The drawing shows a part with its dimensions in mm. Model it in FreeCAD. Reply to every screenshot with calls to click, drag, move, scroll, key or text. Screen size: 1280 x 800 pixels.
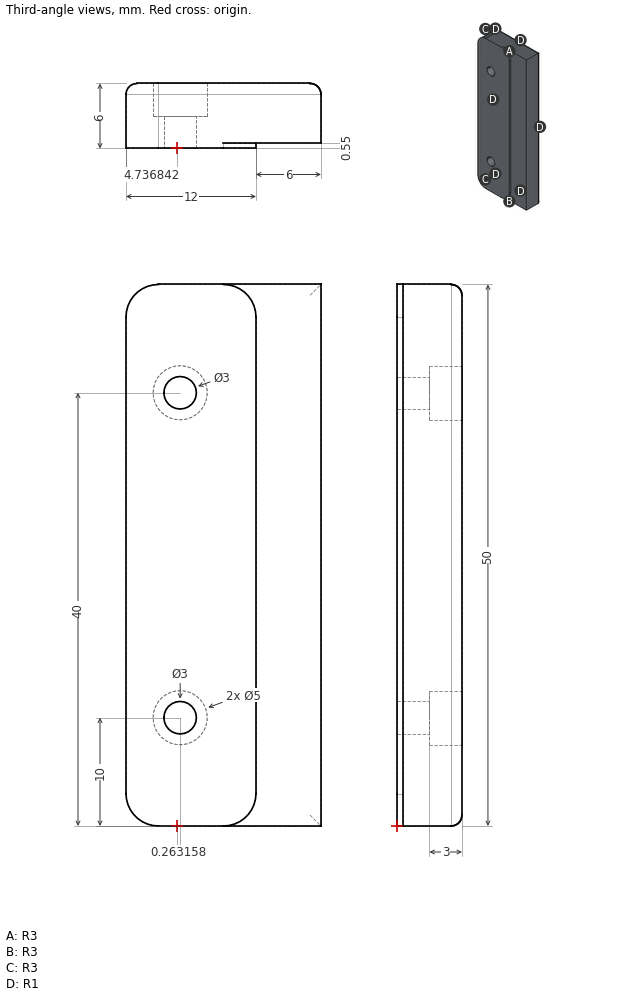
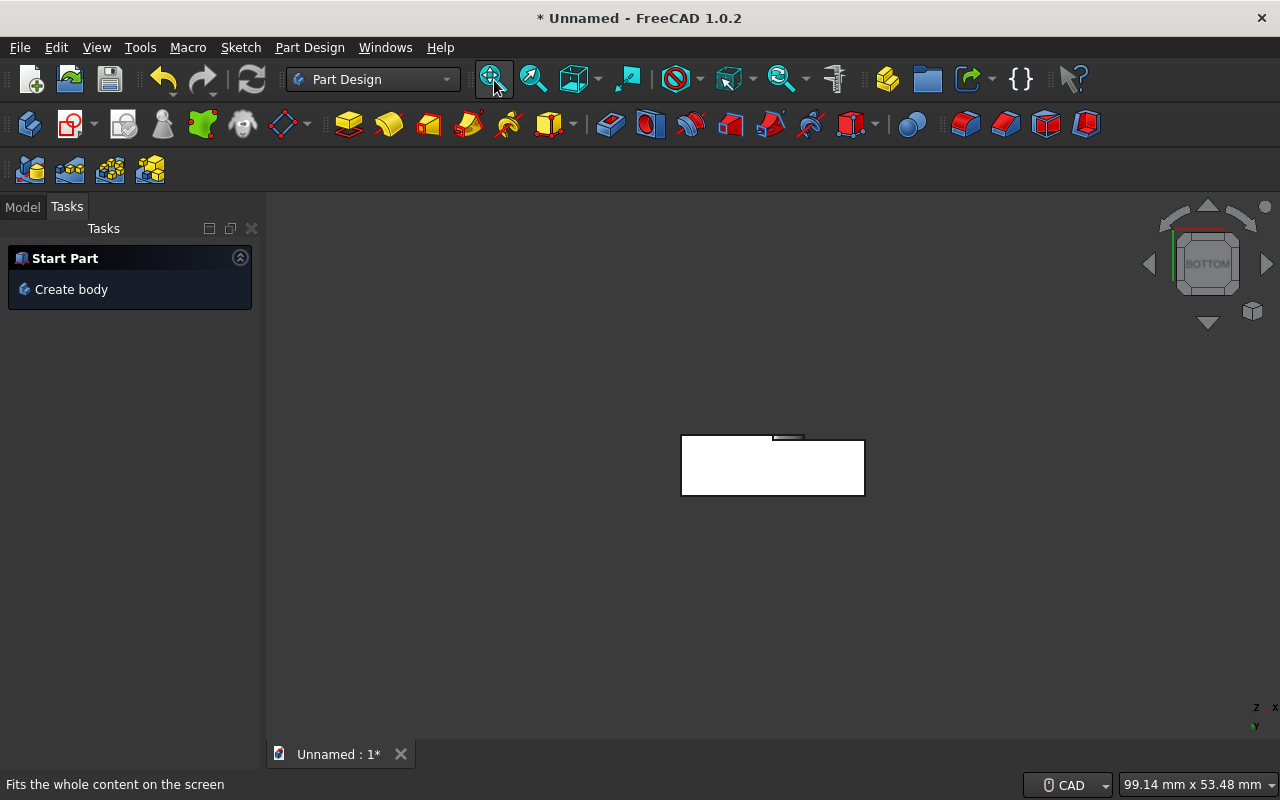
key(0)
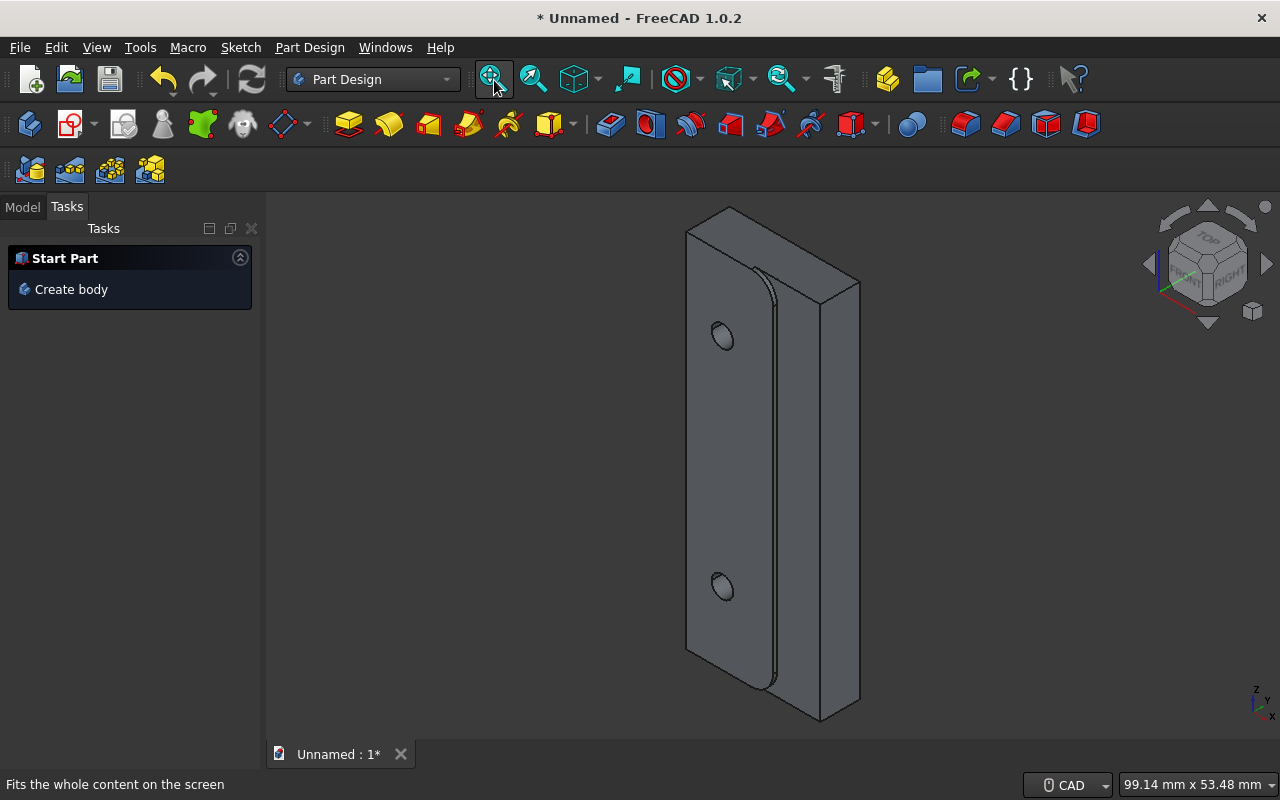
key(2)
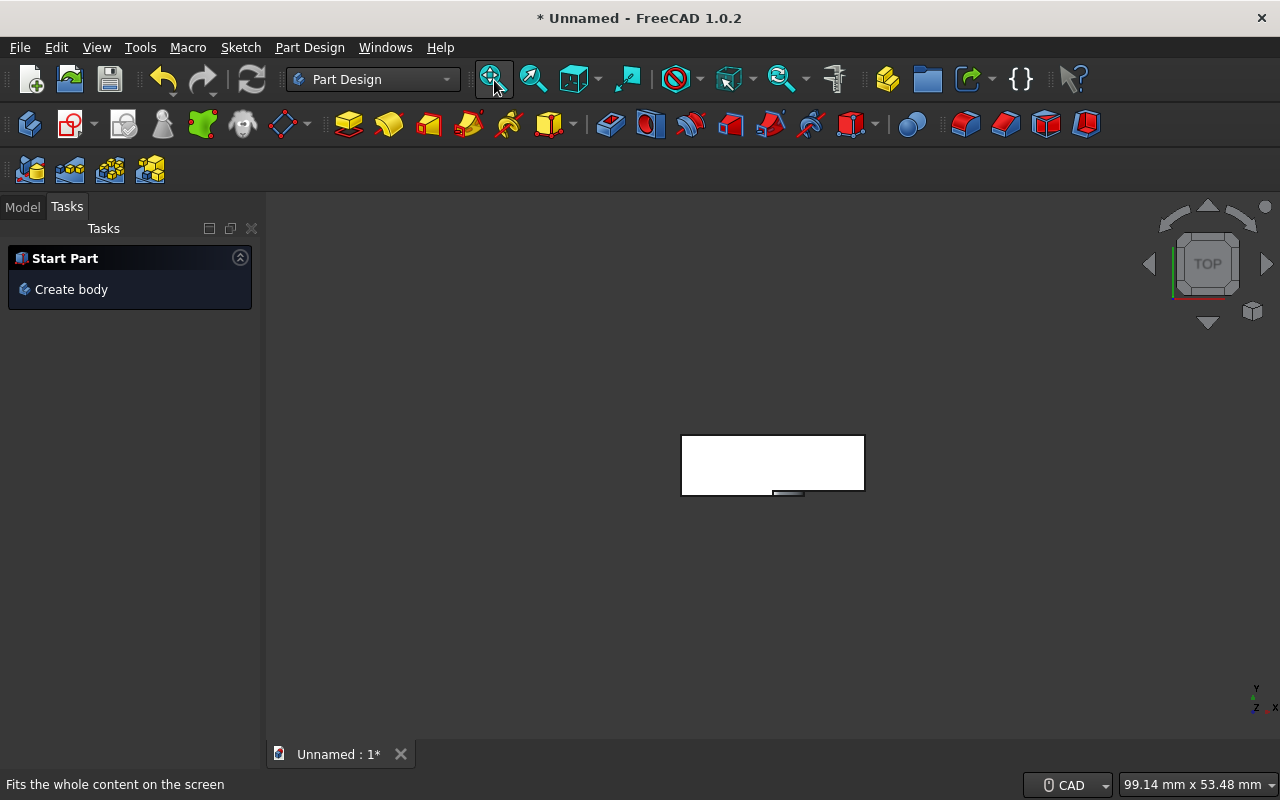
click(494, 80)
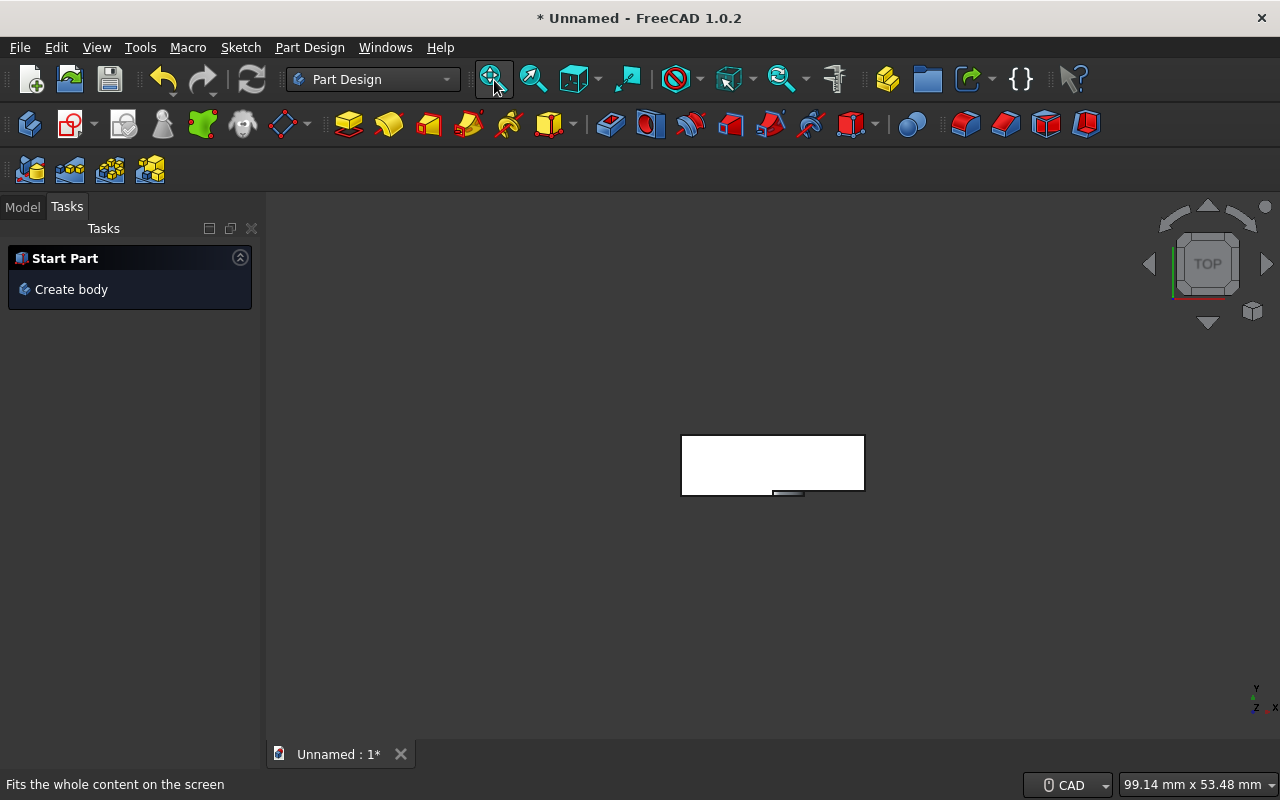
click(681, 464)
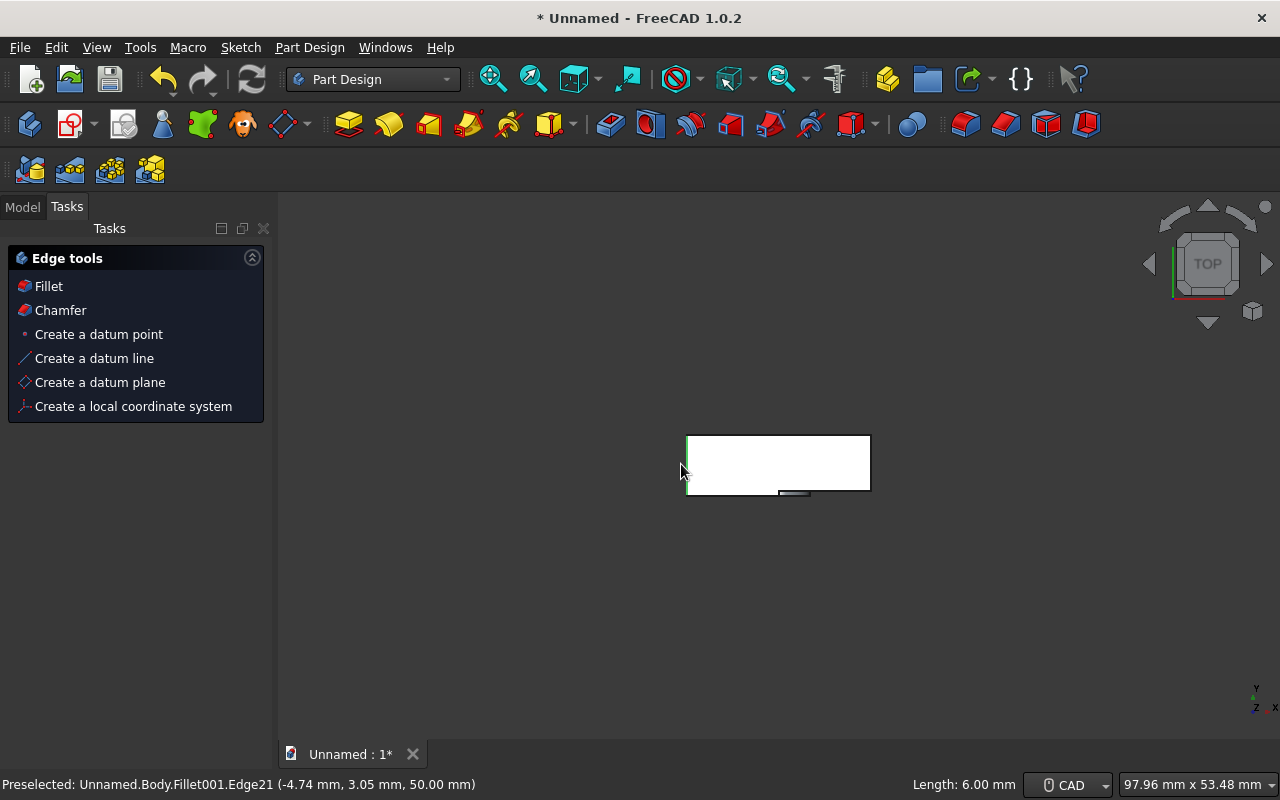
key(1)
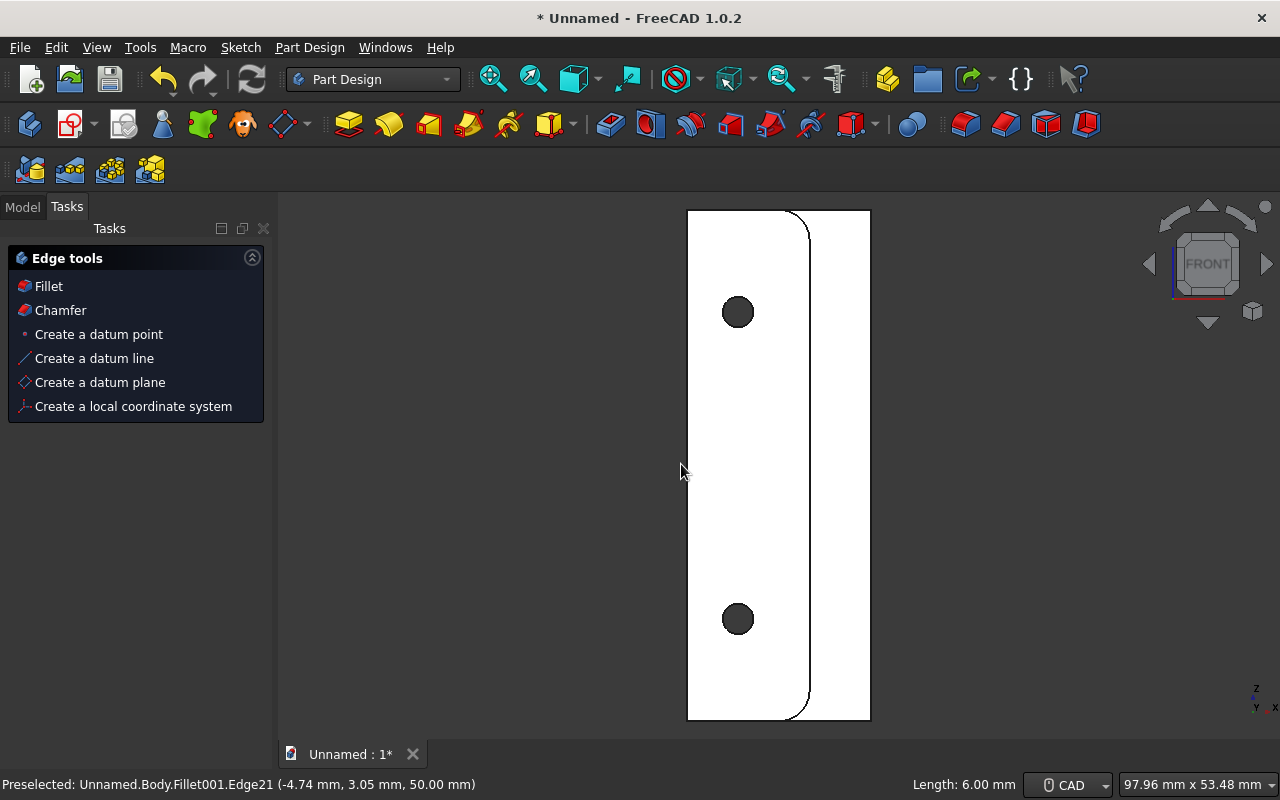
key(3)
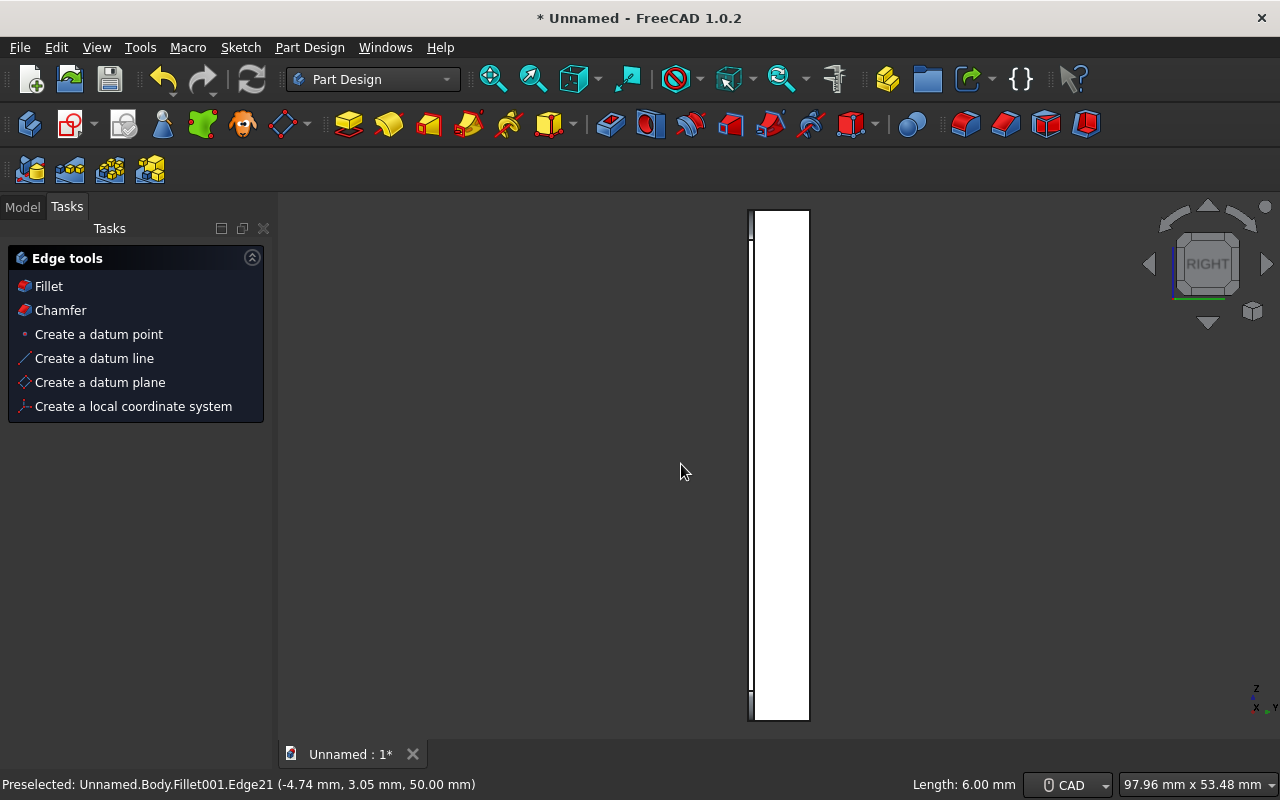
key(5)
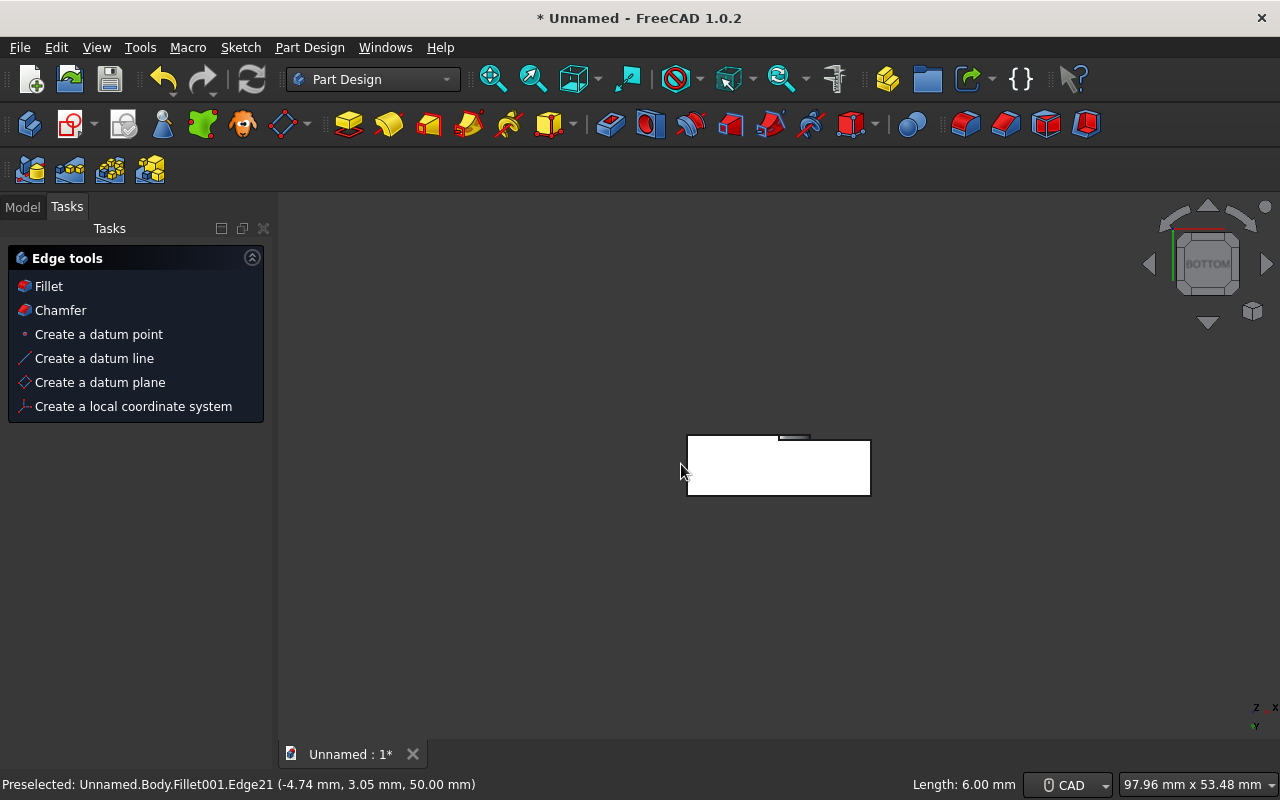
click(494, 80)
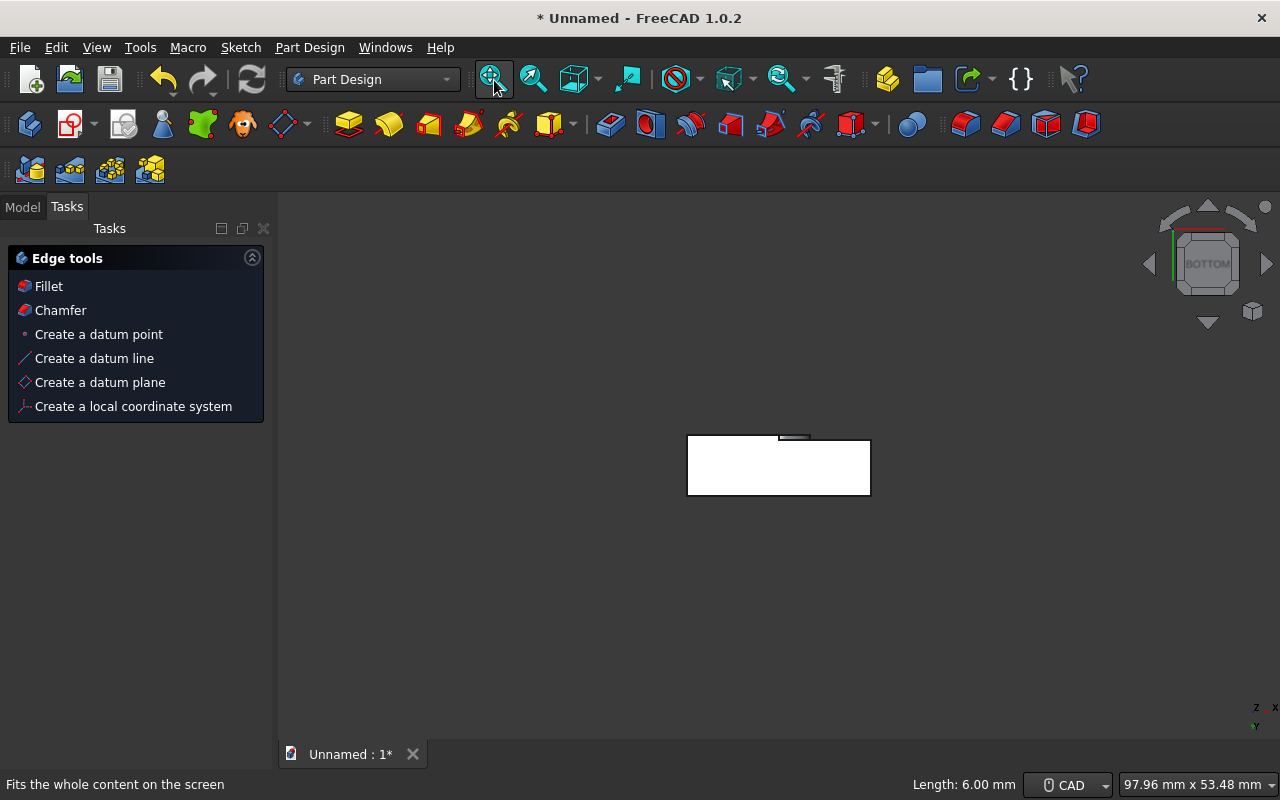
key(4)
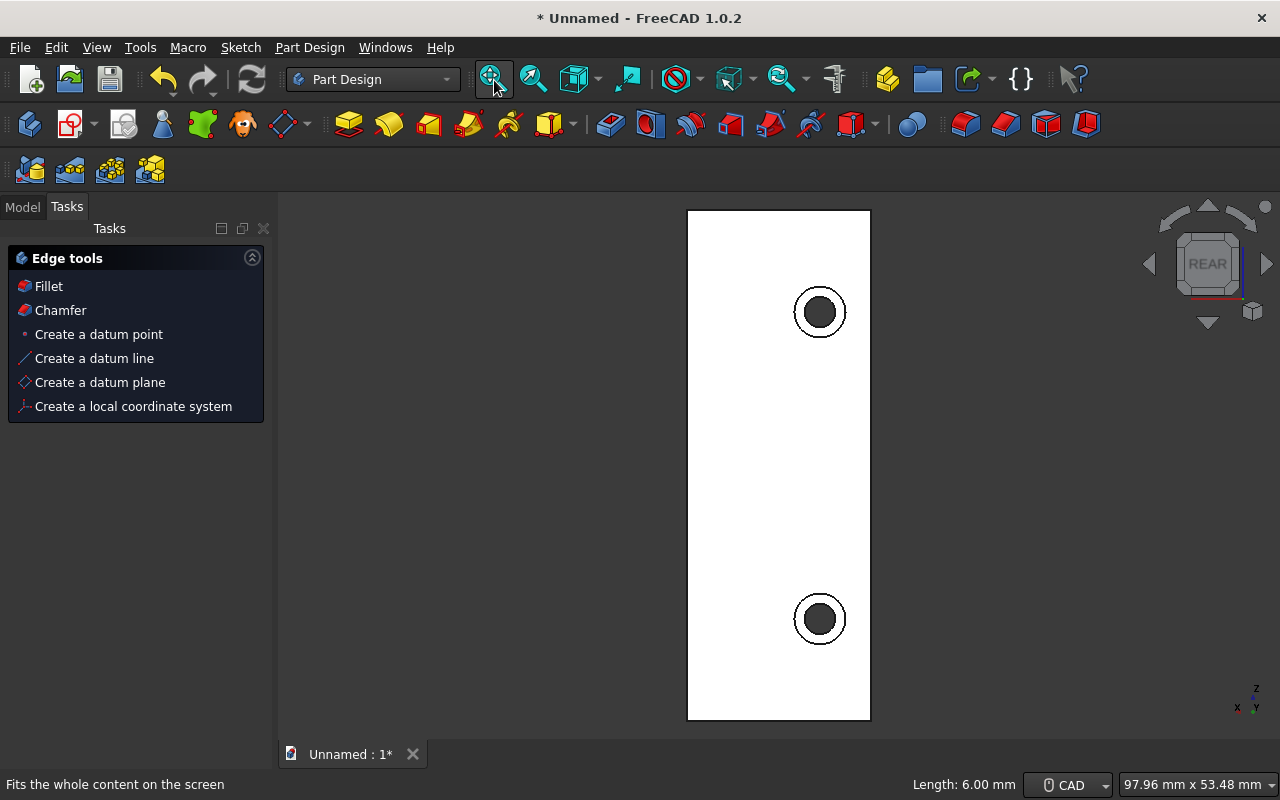
key(6)